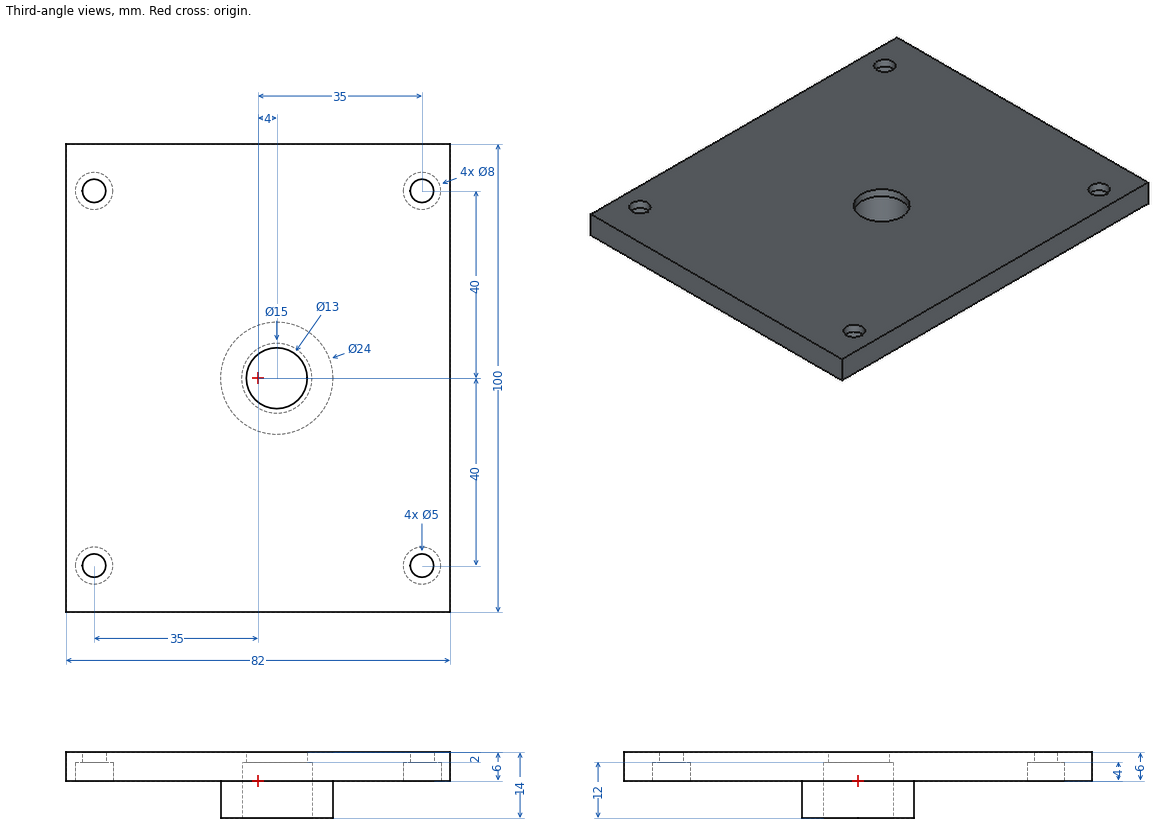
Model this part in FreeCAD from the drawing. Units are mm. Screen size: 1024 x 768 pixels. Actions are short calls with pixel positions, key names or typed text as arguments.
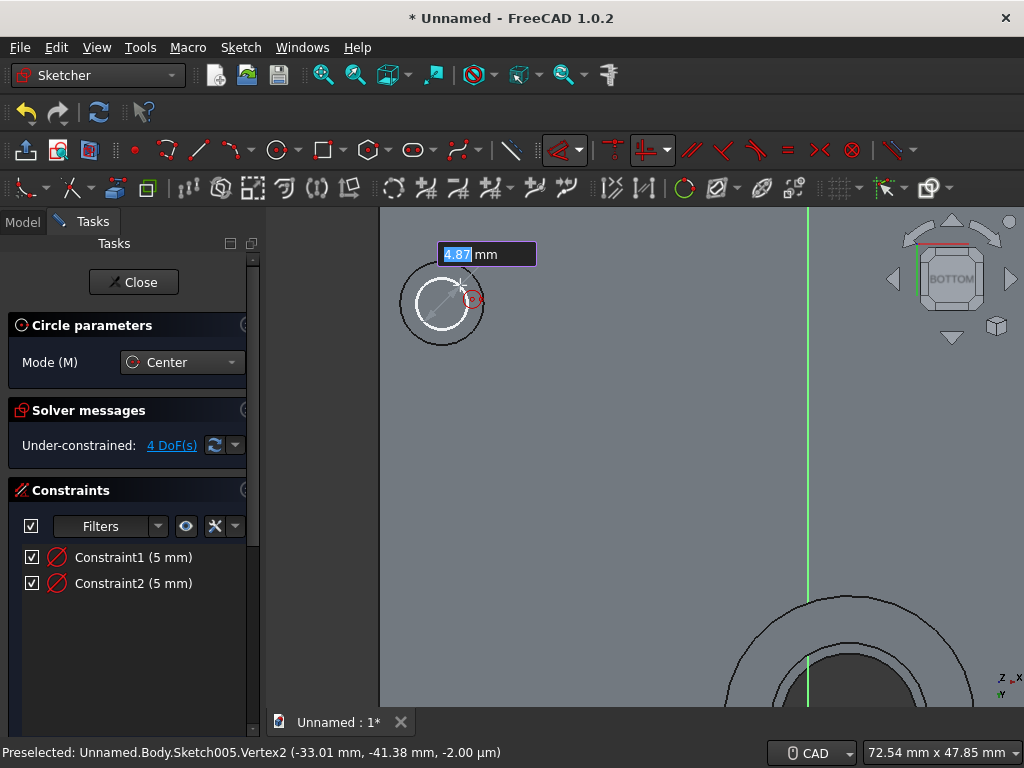
text(5)
key(Return)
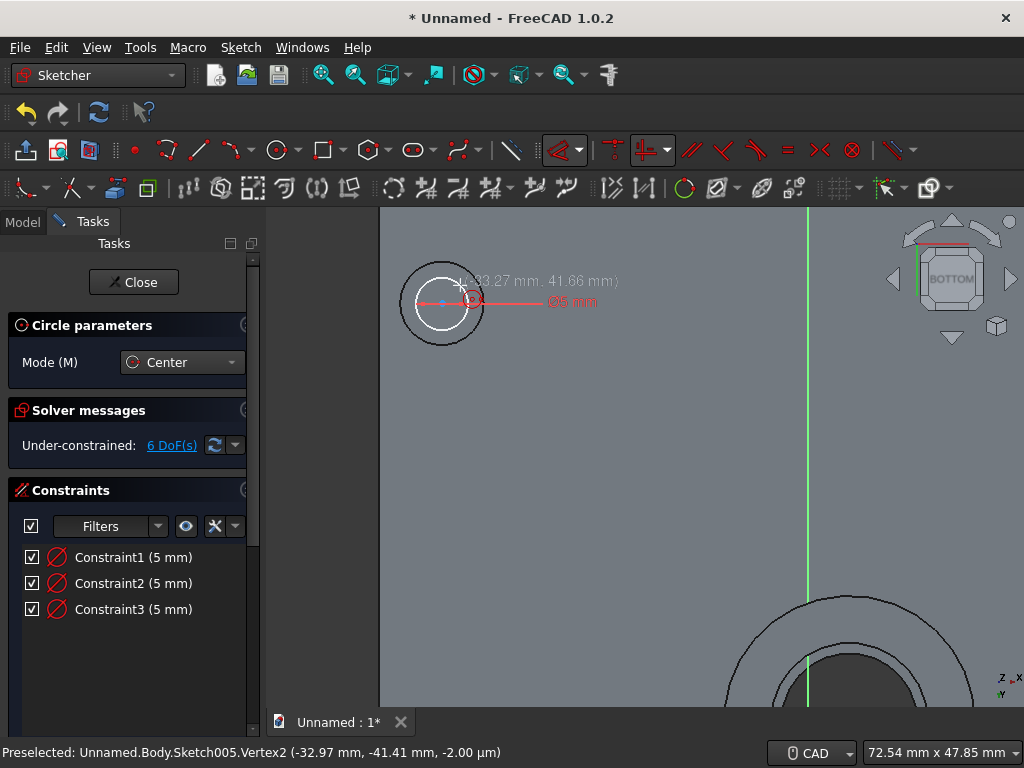
scroll(442, 303, down, 5)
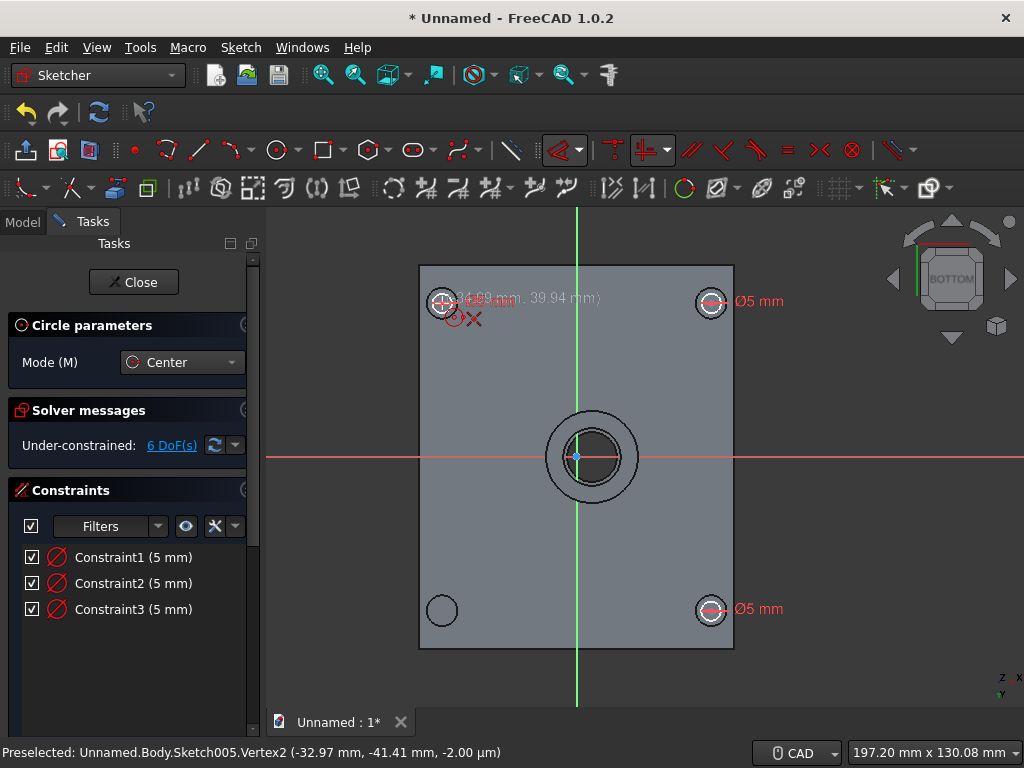
scroll(442, 611, up, 5)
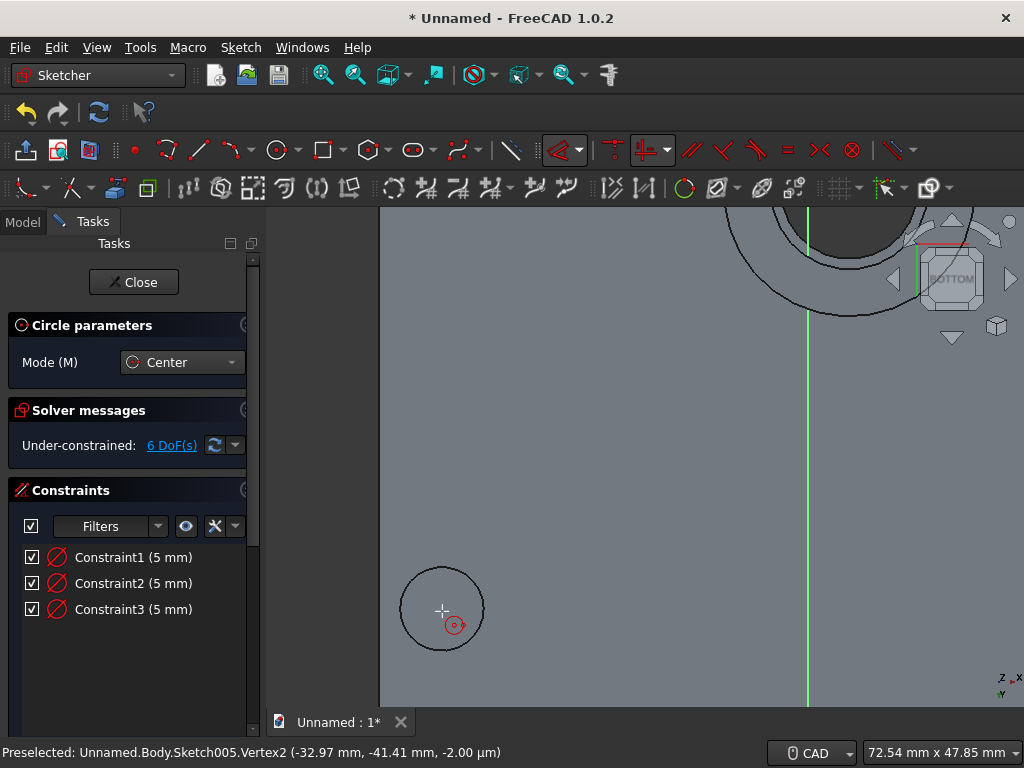
click(442, 609)
move(460, 590)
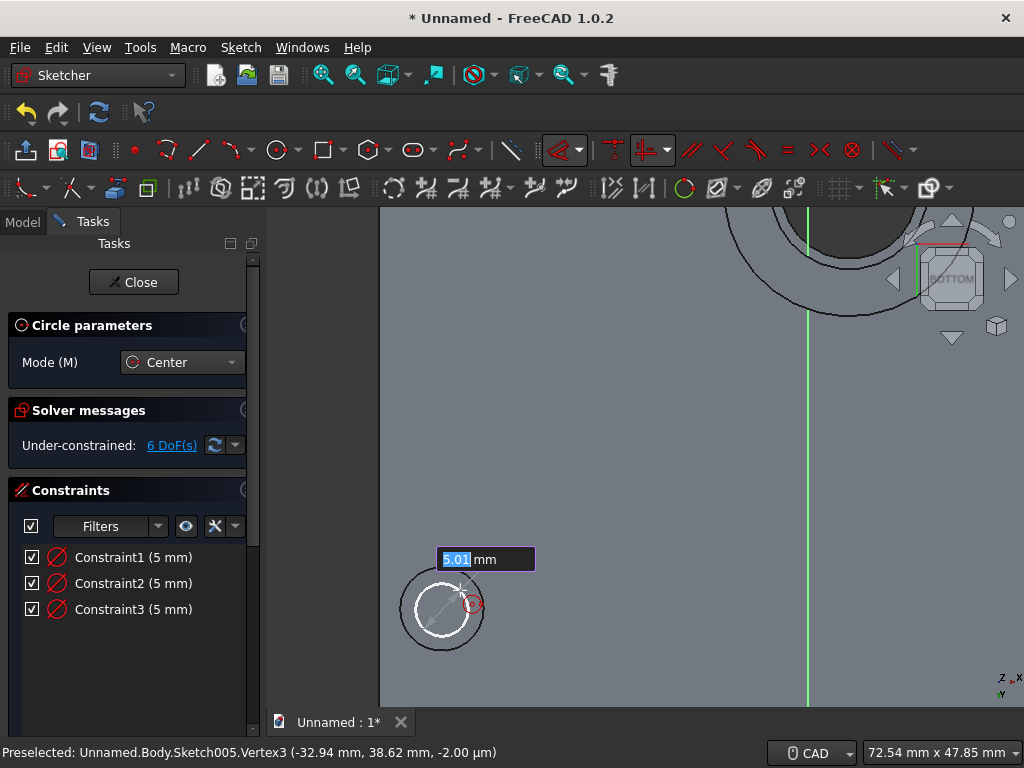
text(5)
key(Return)
key(Escape)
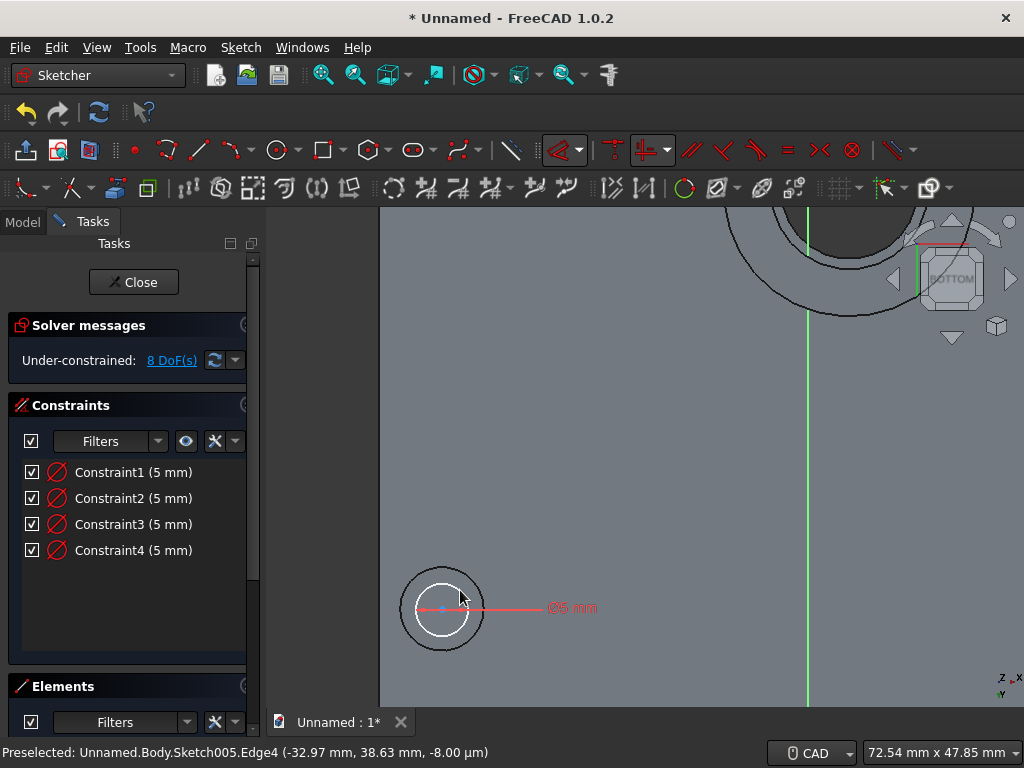
scroll(442, 612, down, 5)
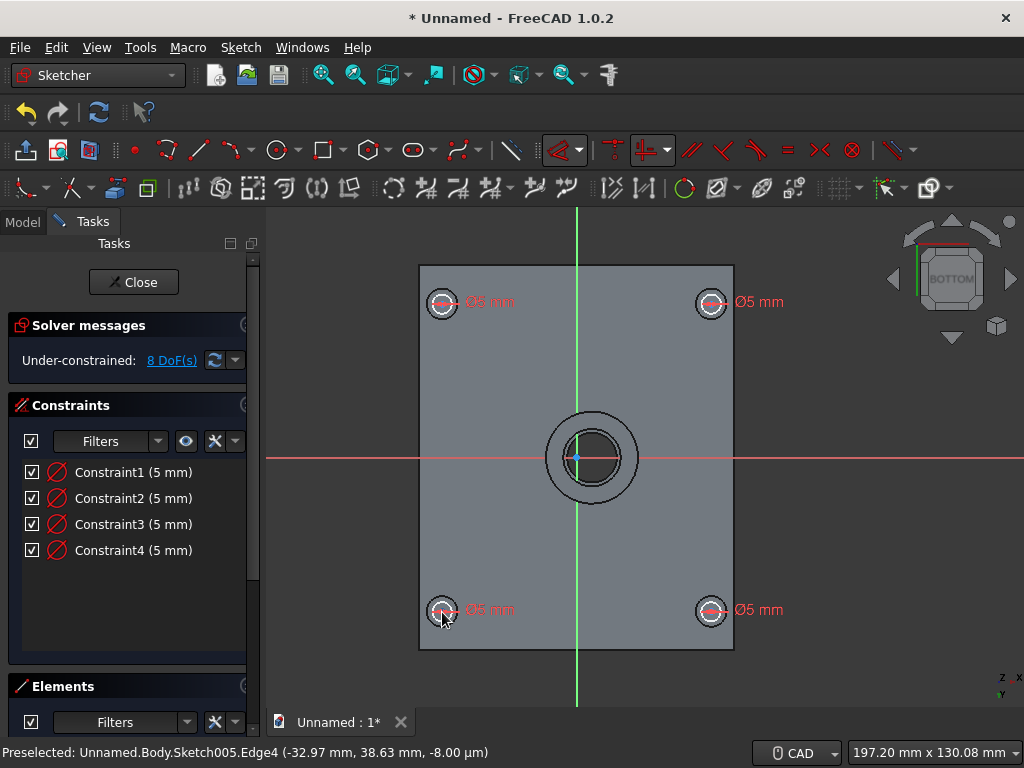
click(711, 304)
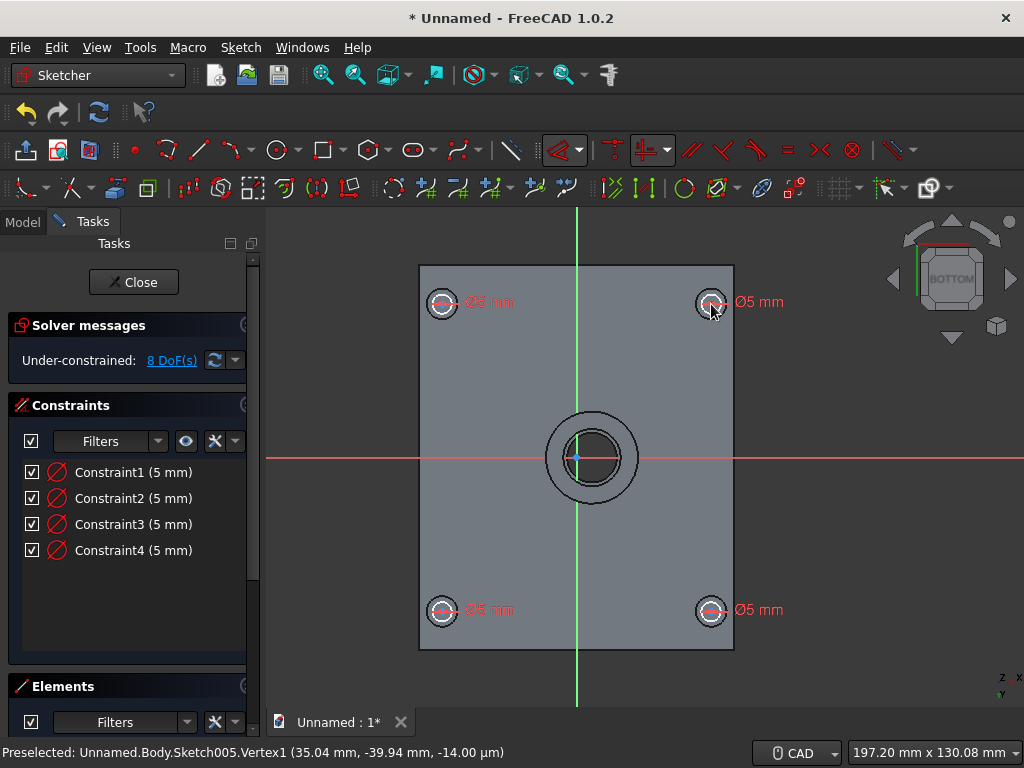
click(711, 612)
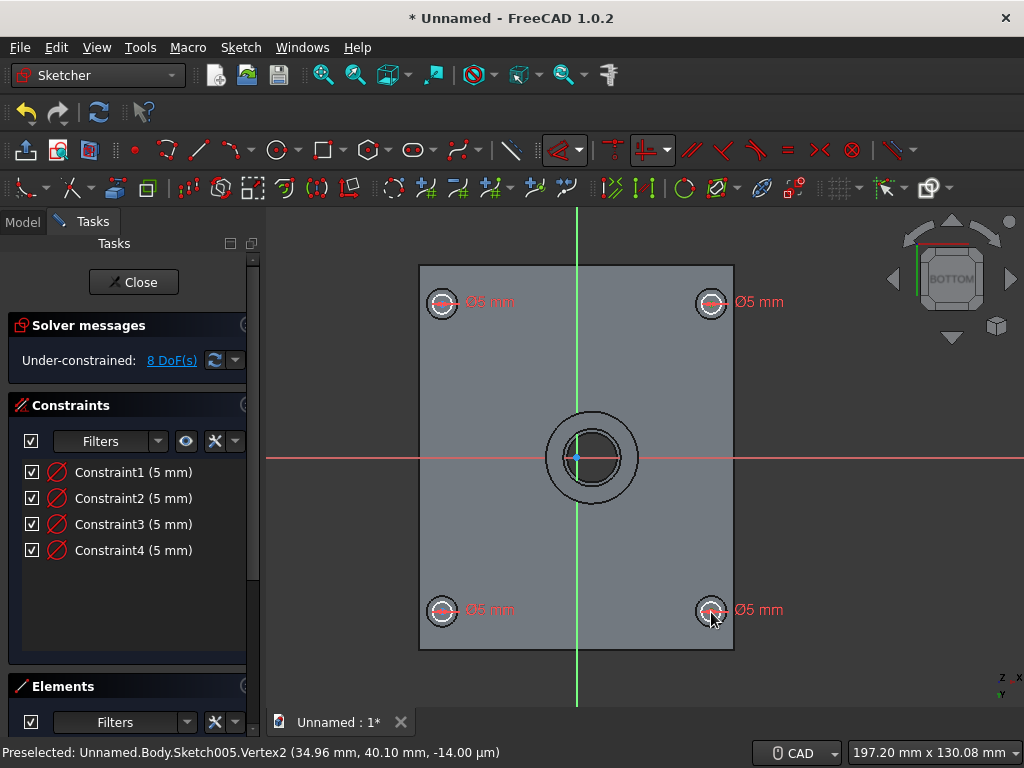
key(v)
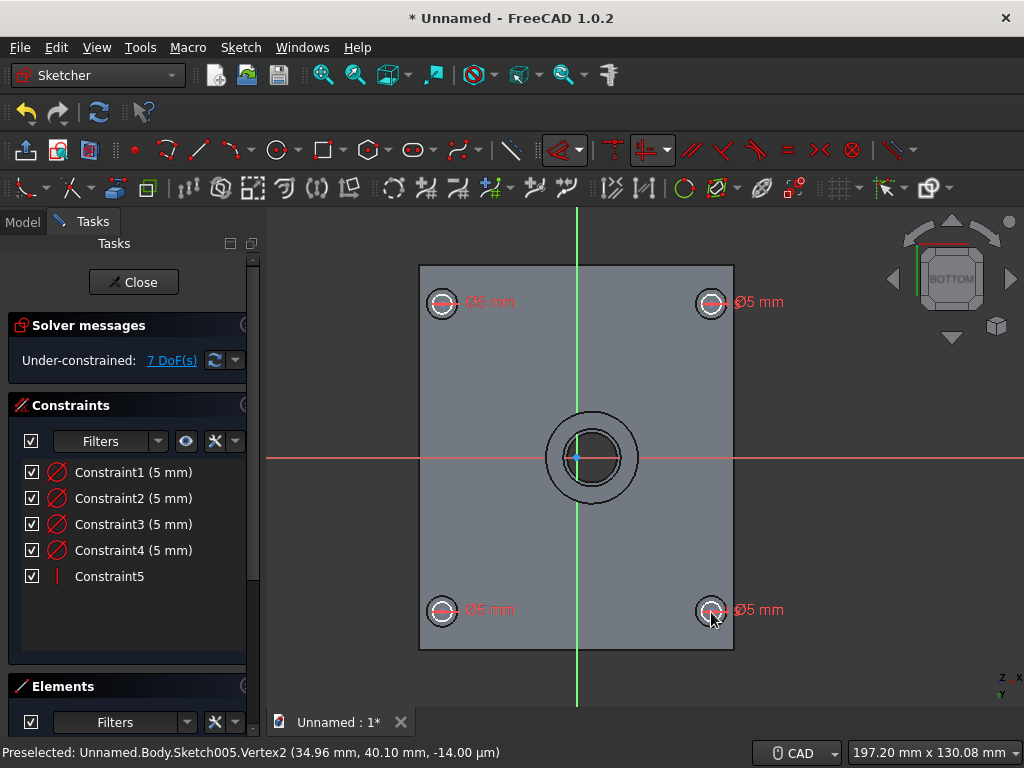
click(711, 304)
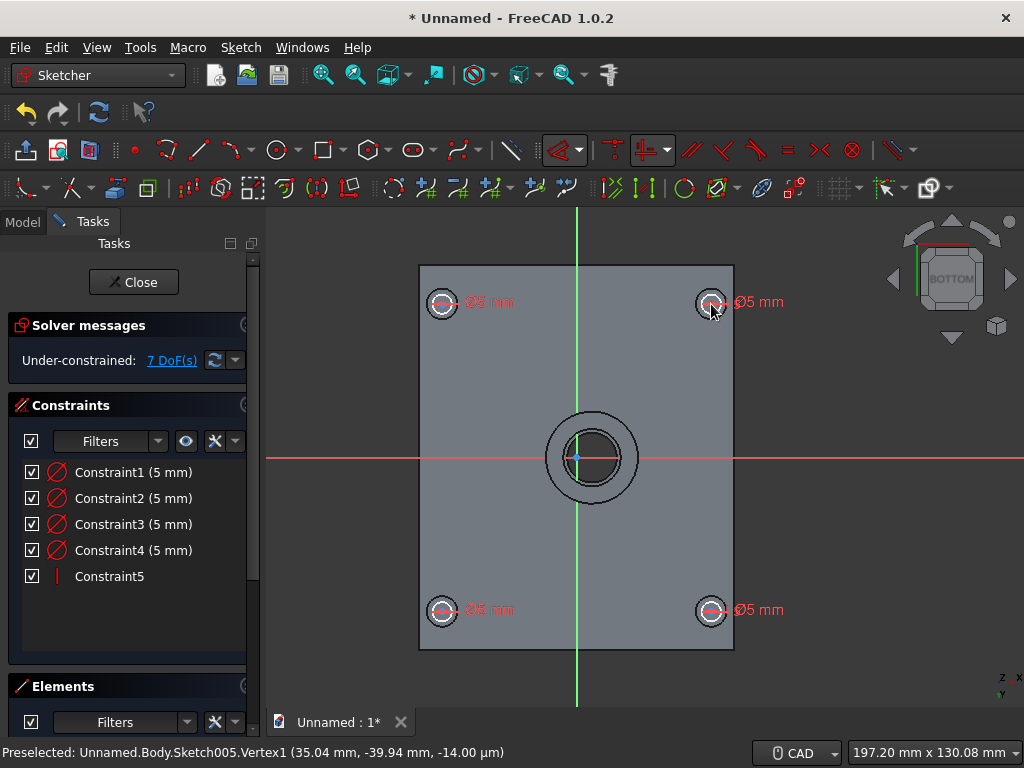
click(442, 304)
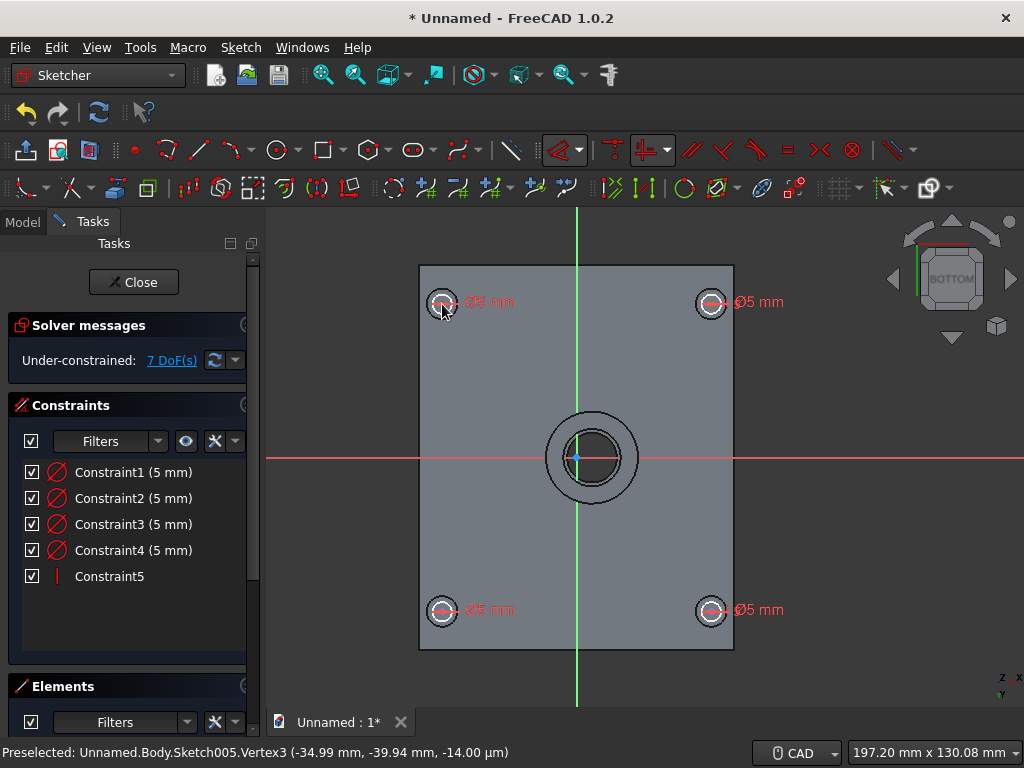
key(h)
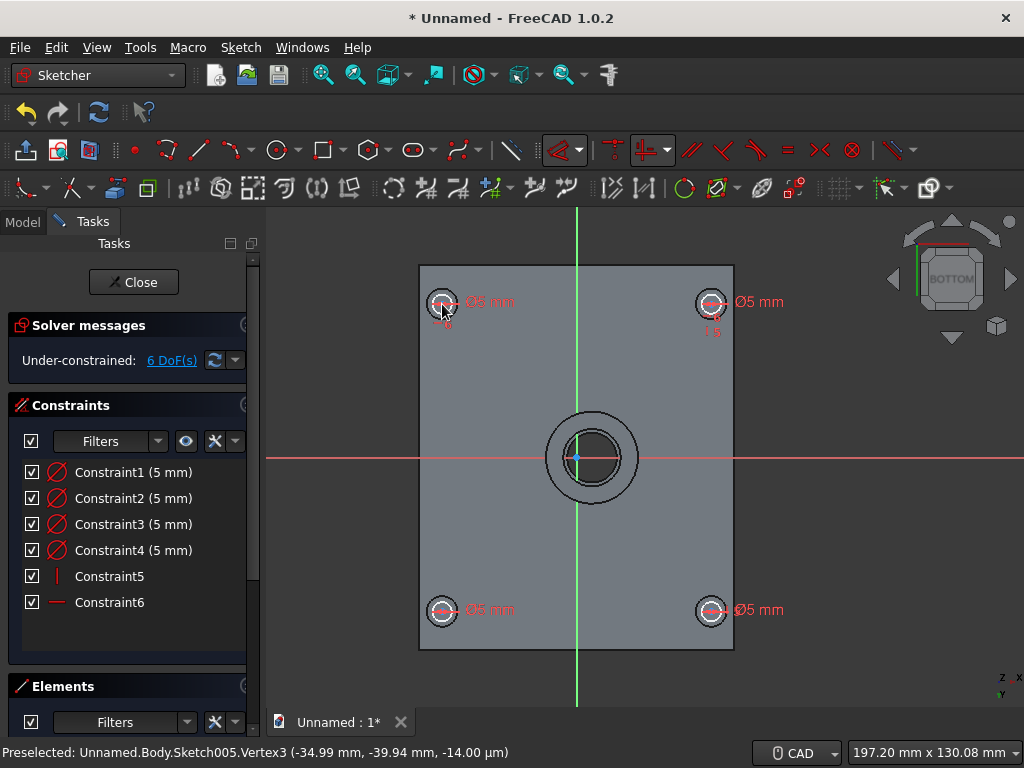
click(442, 304)